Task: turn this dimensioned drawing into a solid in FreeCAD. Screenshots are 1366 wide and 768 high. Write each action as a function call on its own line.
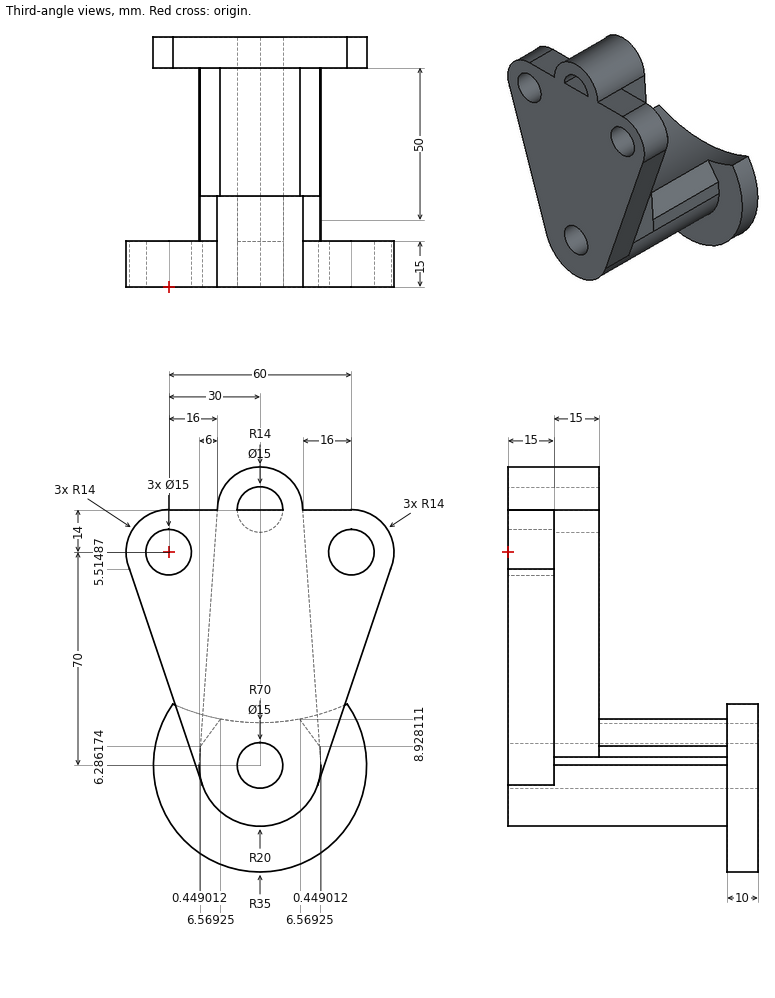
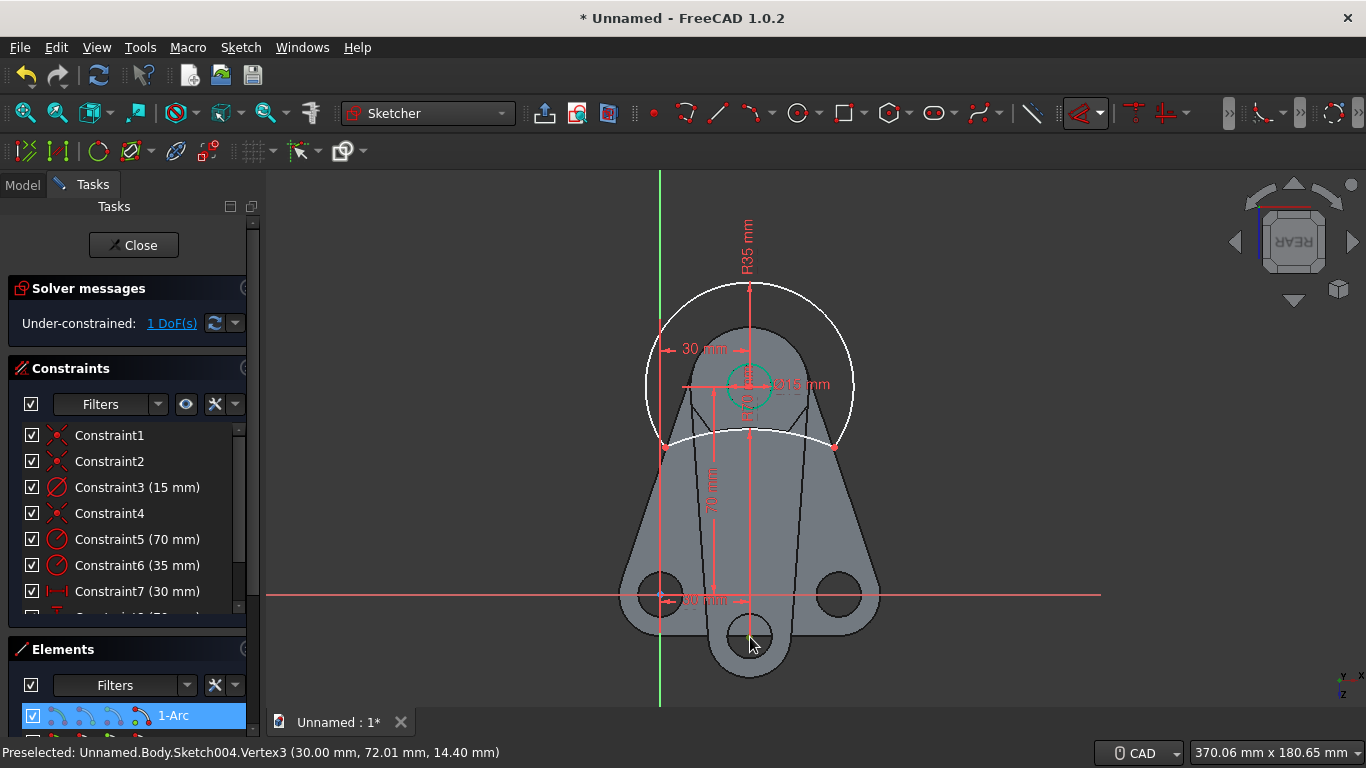
click(1102, 114)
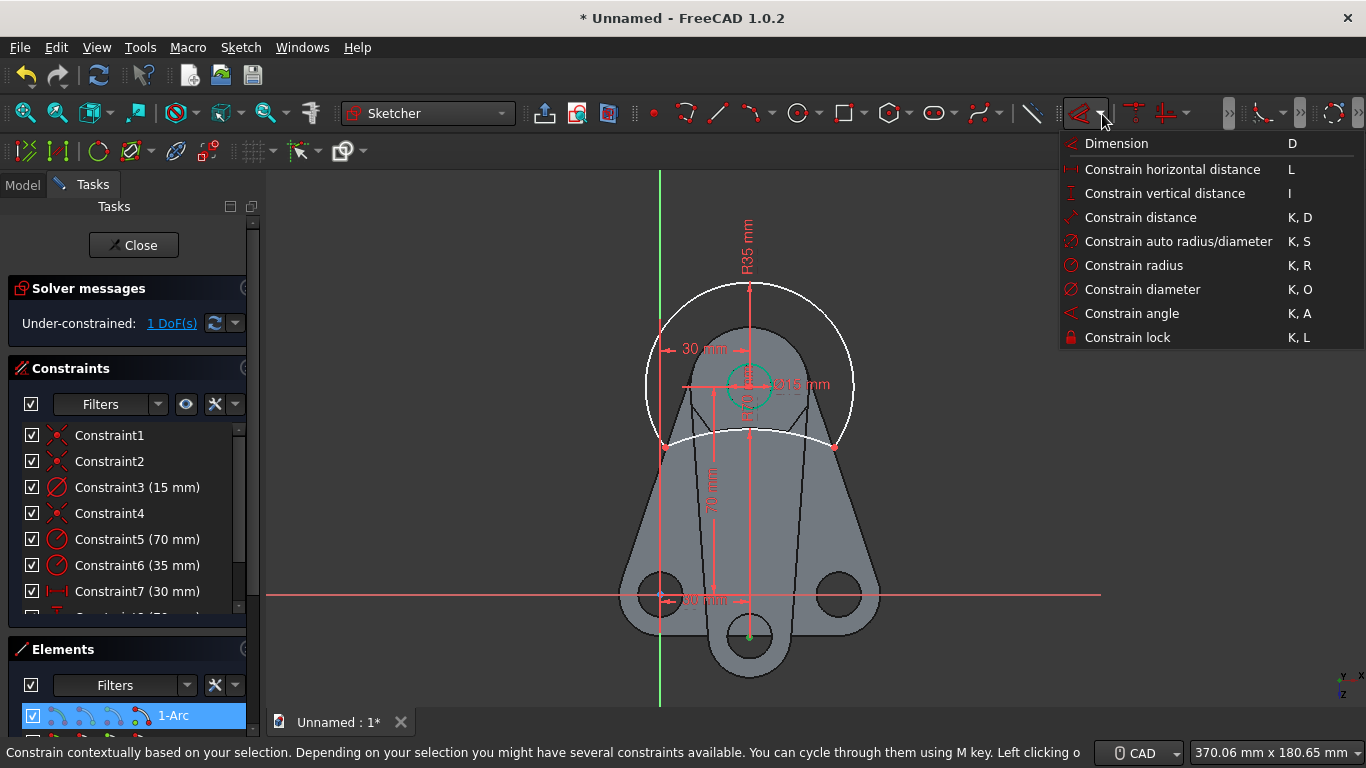
click(1212, 193)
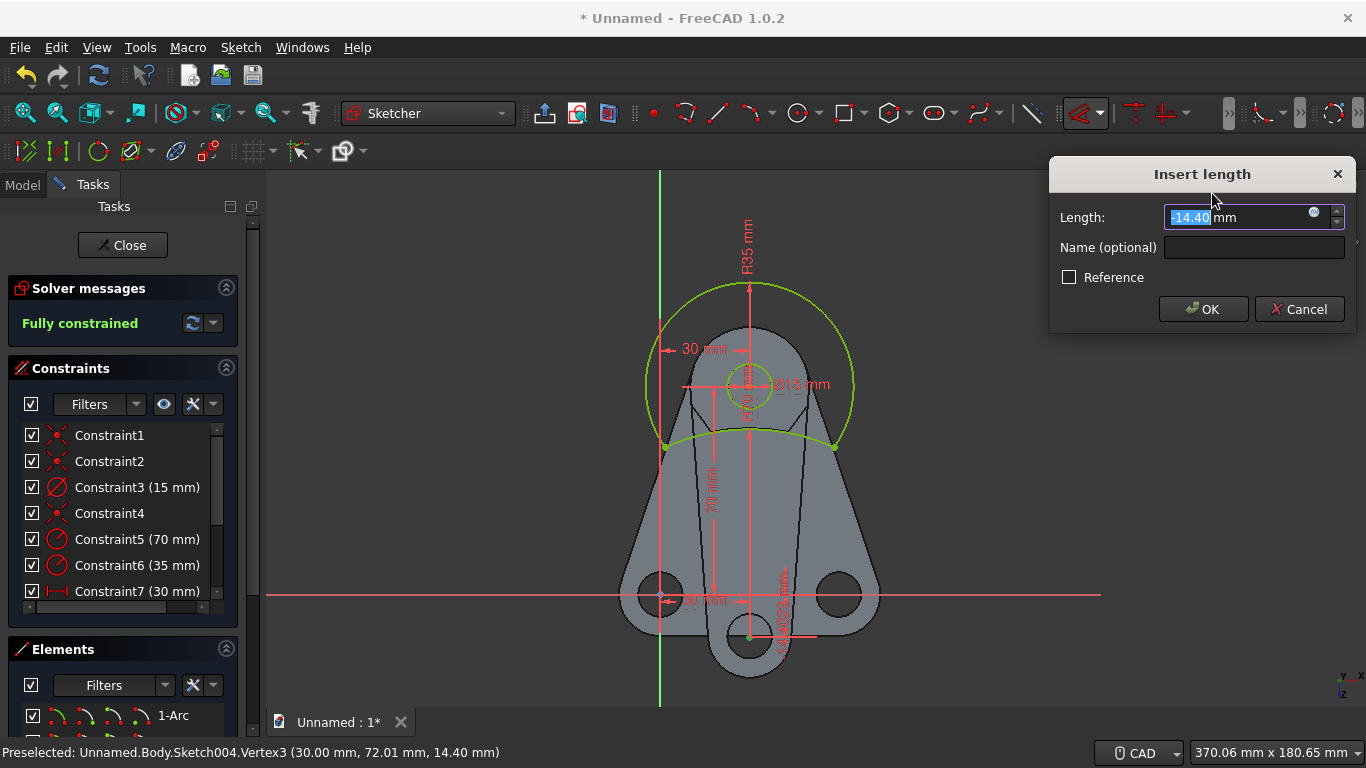
text(-14)
key(Return)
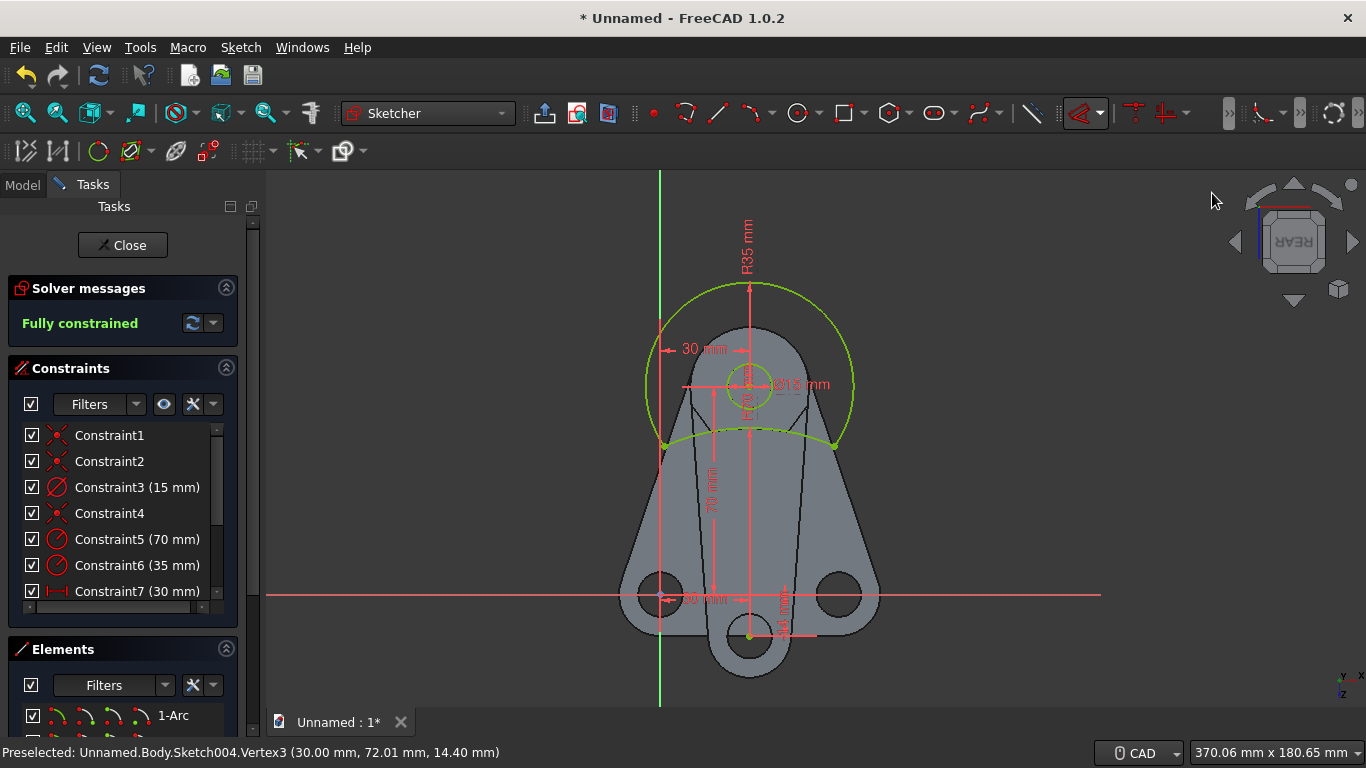
click(123, 245)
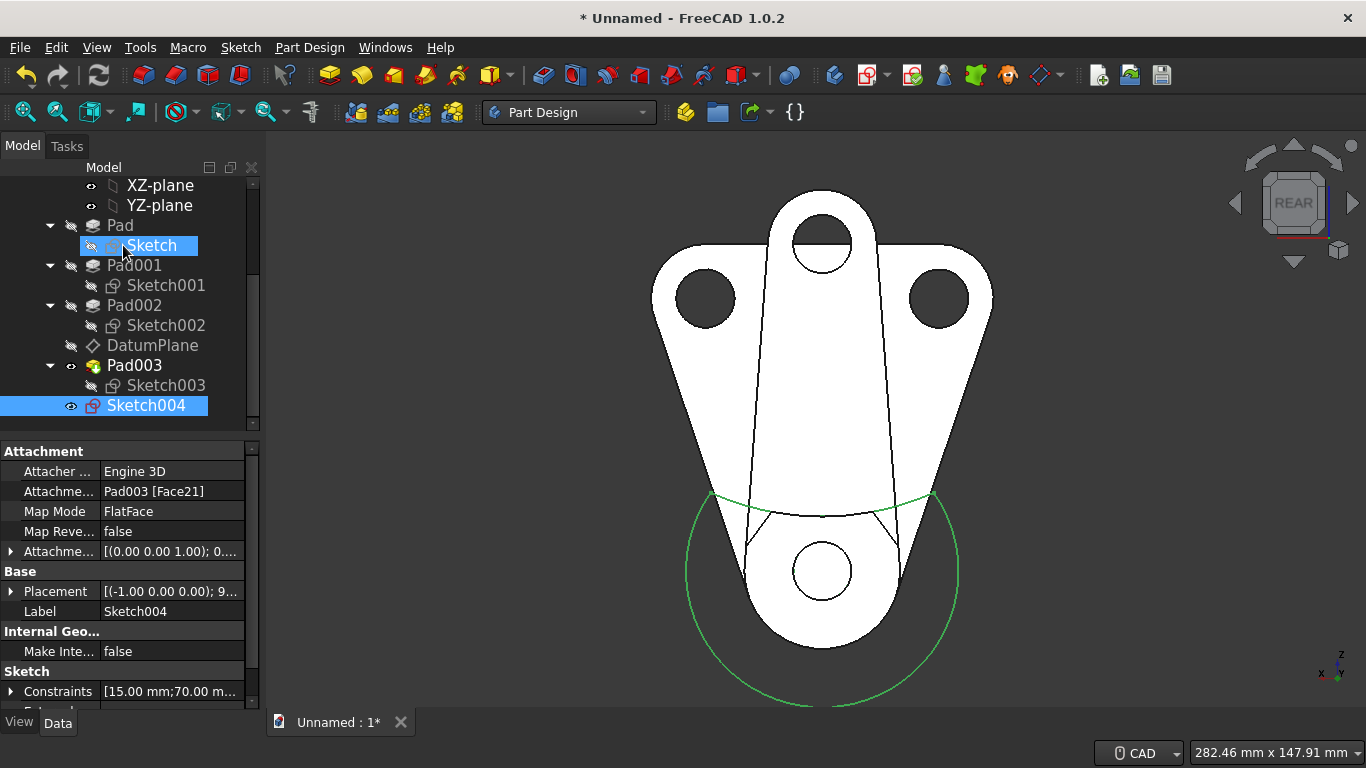
click(330, 76)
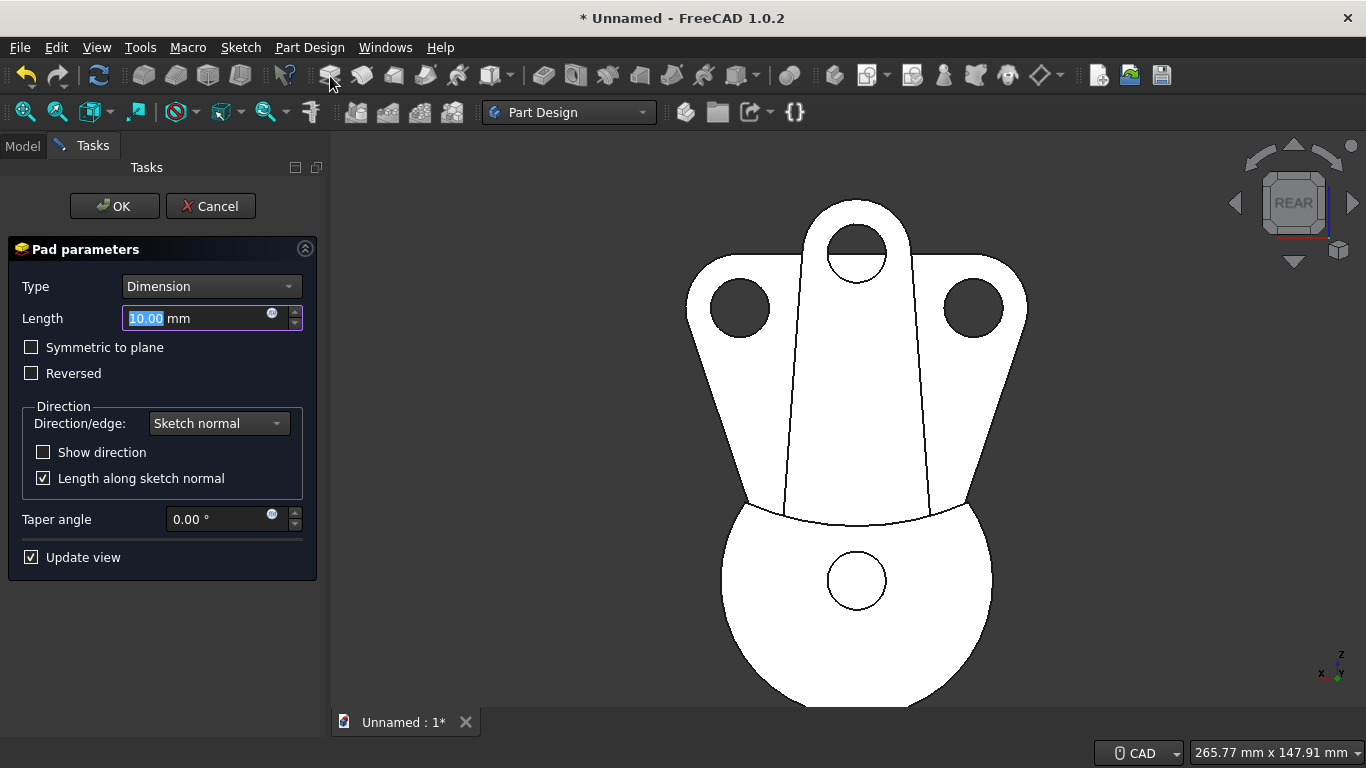
text(10)
key(Tab)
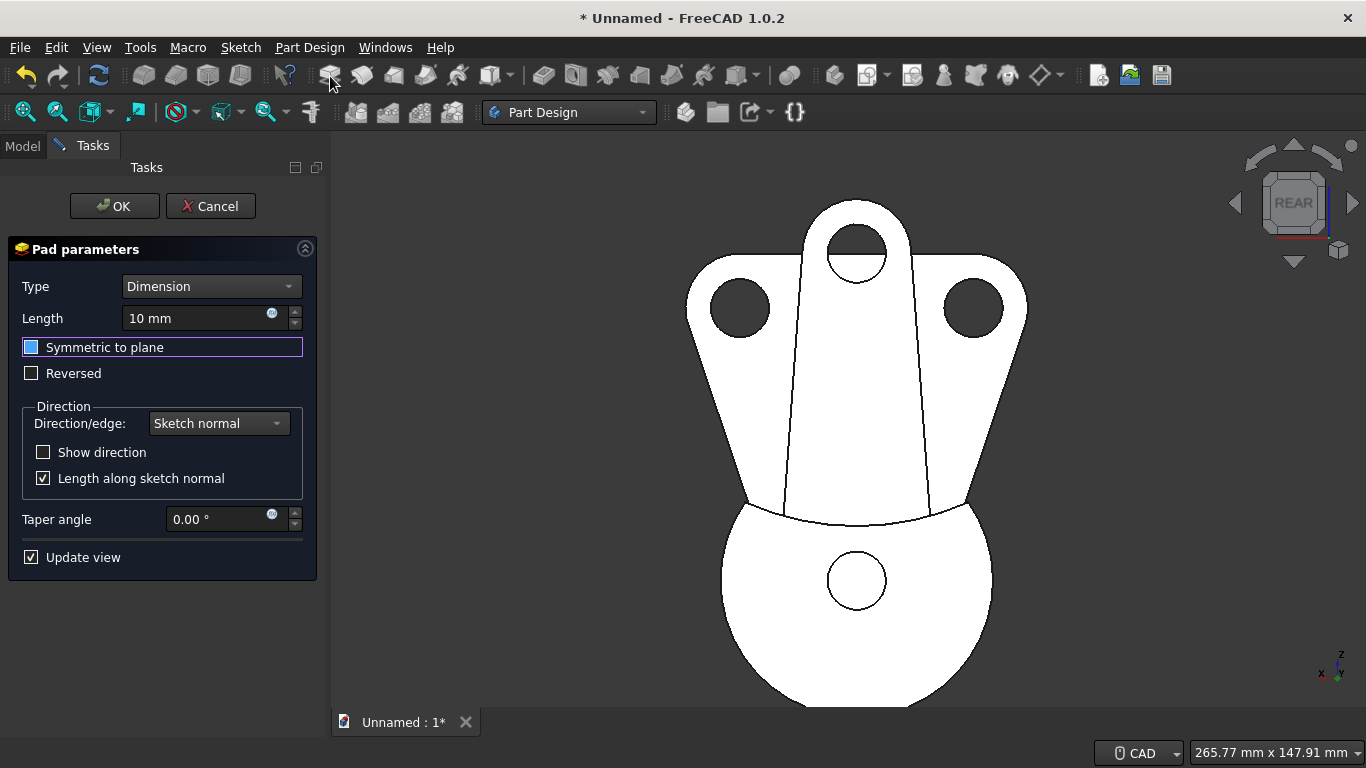
click(115, 206)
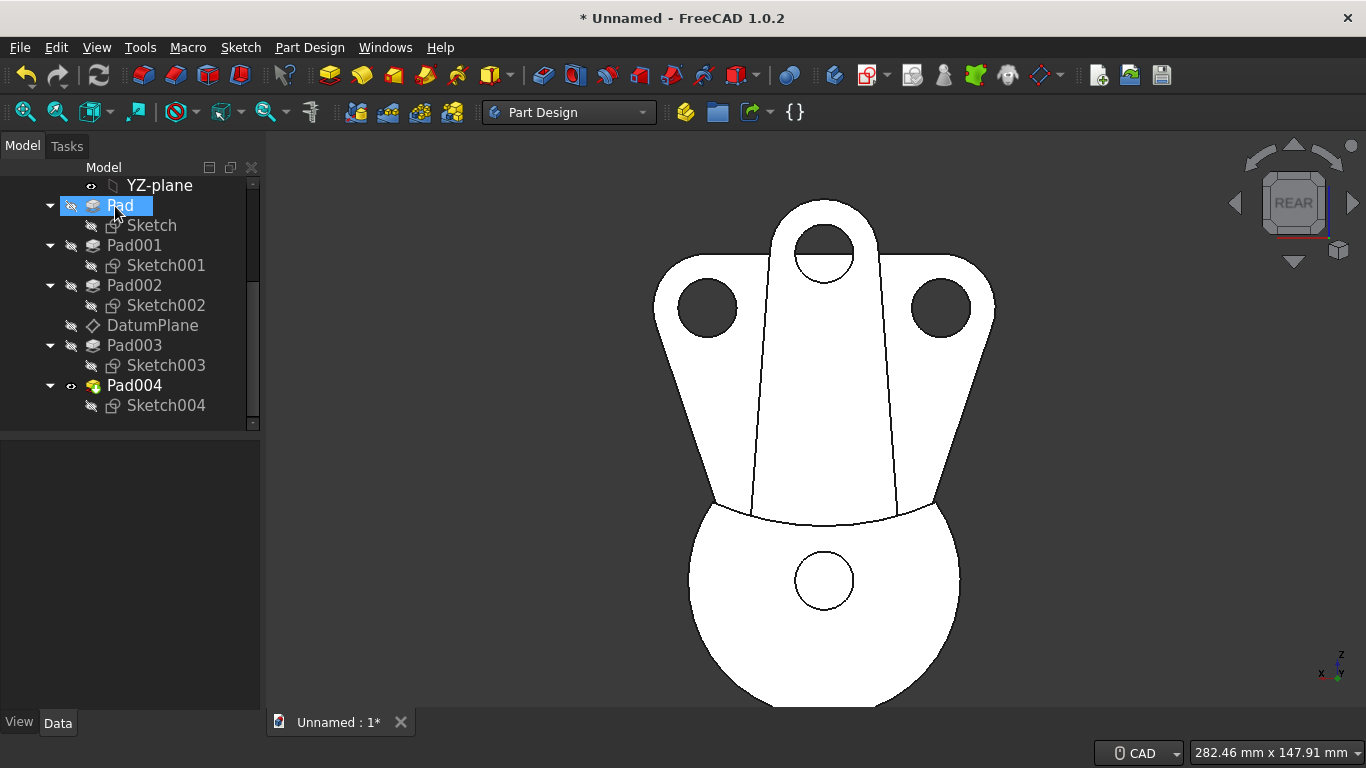
click(26, 112)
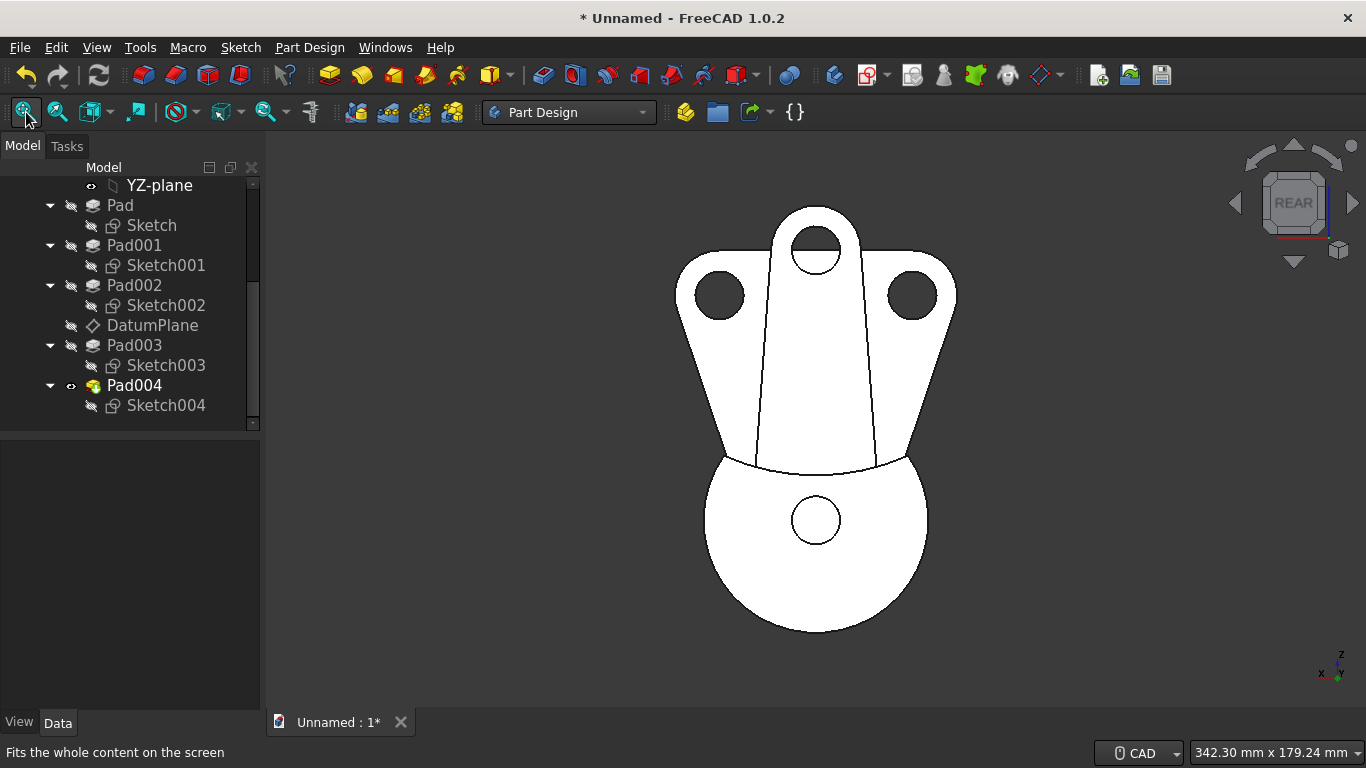
scroll(160, 301, down, 3)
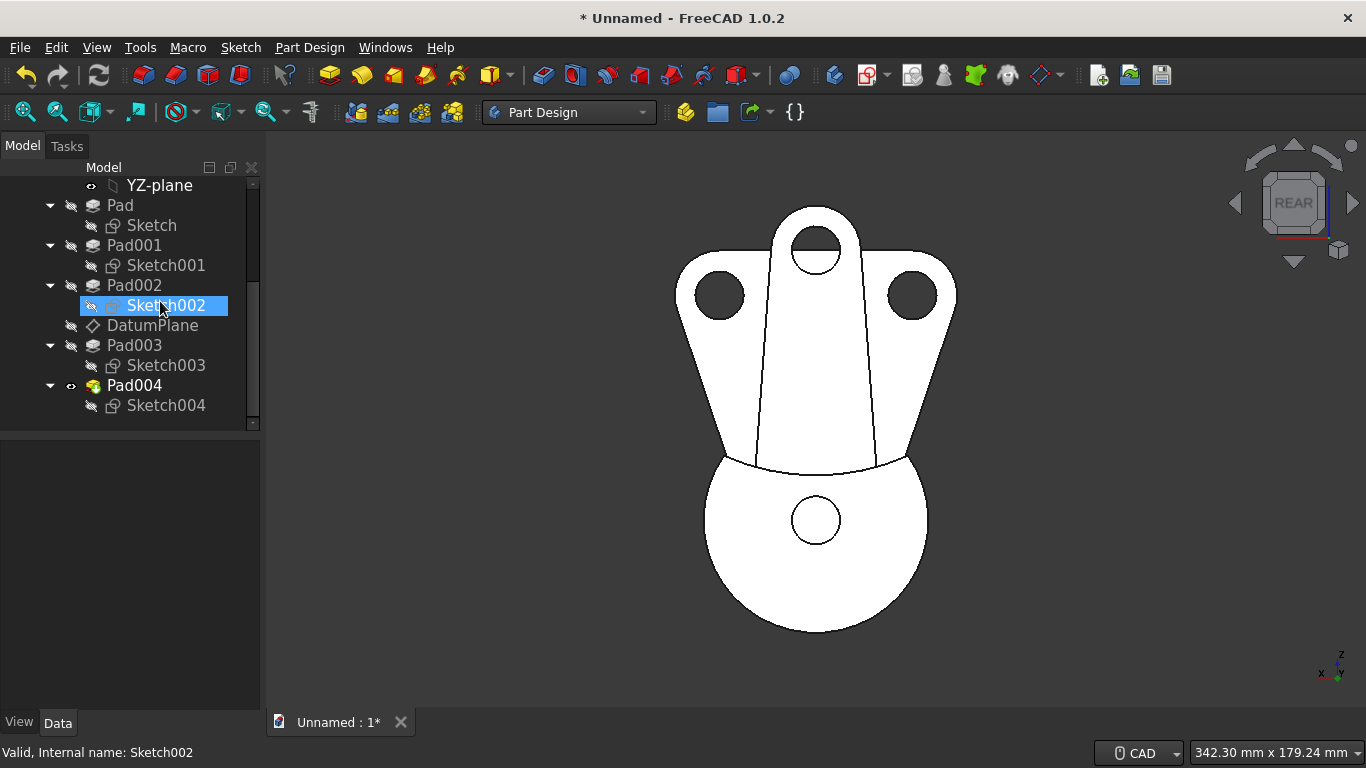
scroll(160, 301, up, 15)